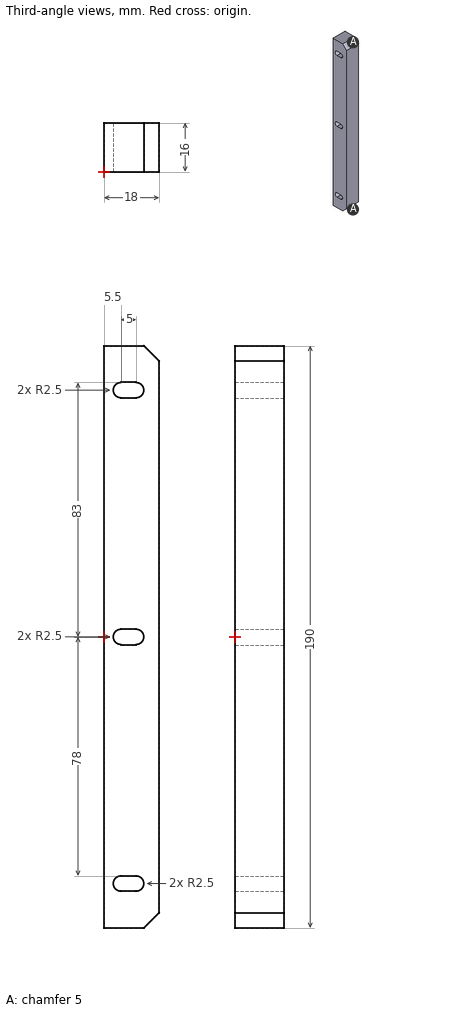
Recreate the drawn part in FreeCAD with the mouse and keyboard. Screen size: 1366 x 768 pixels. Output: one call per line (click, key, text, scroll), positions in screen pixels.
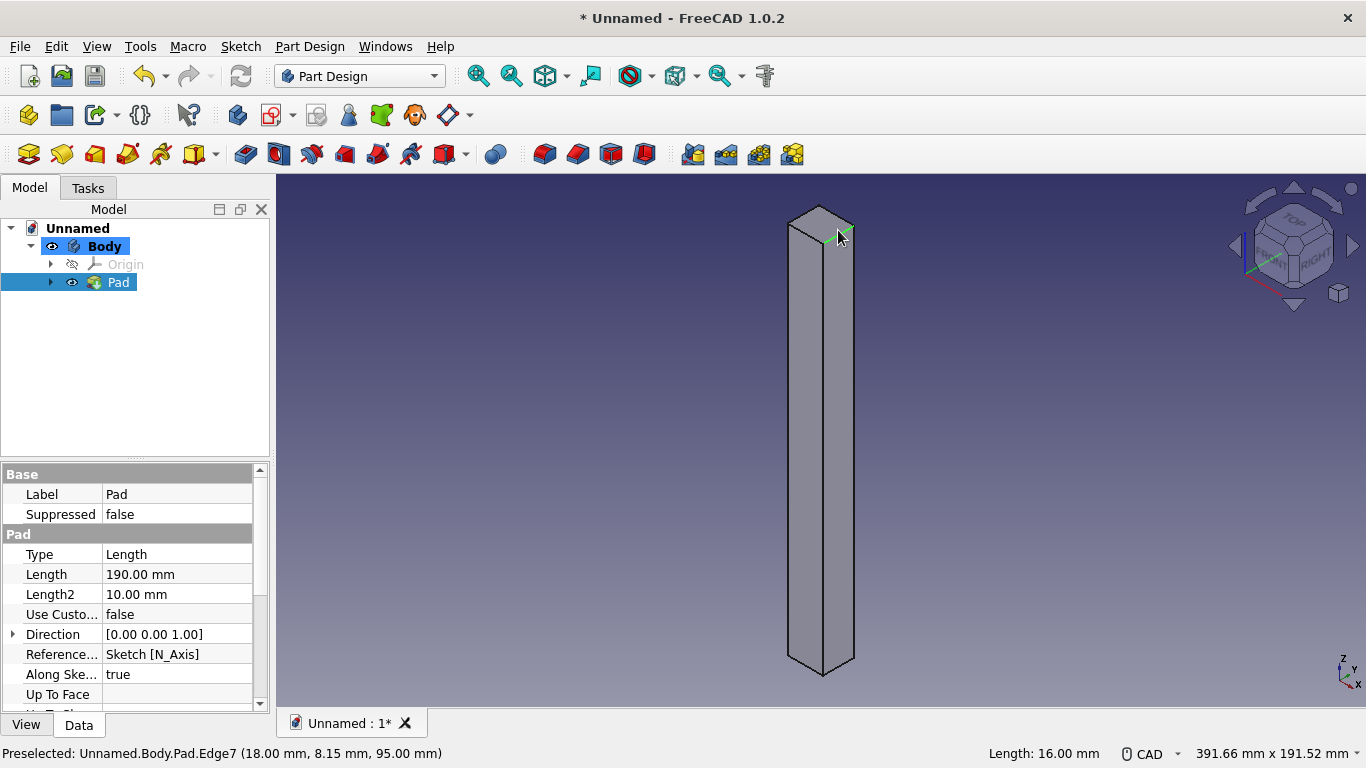
key(2)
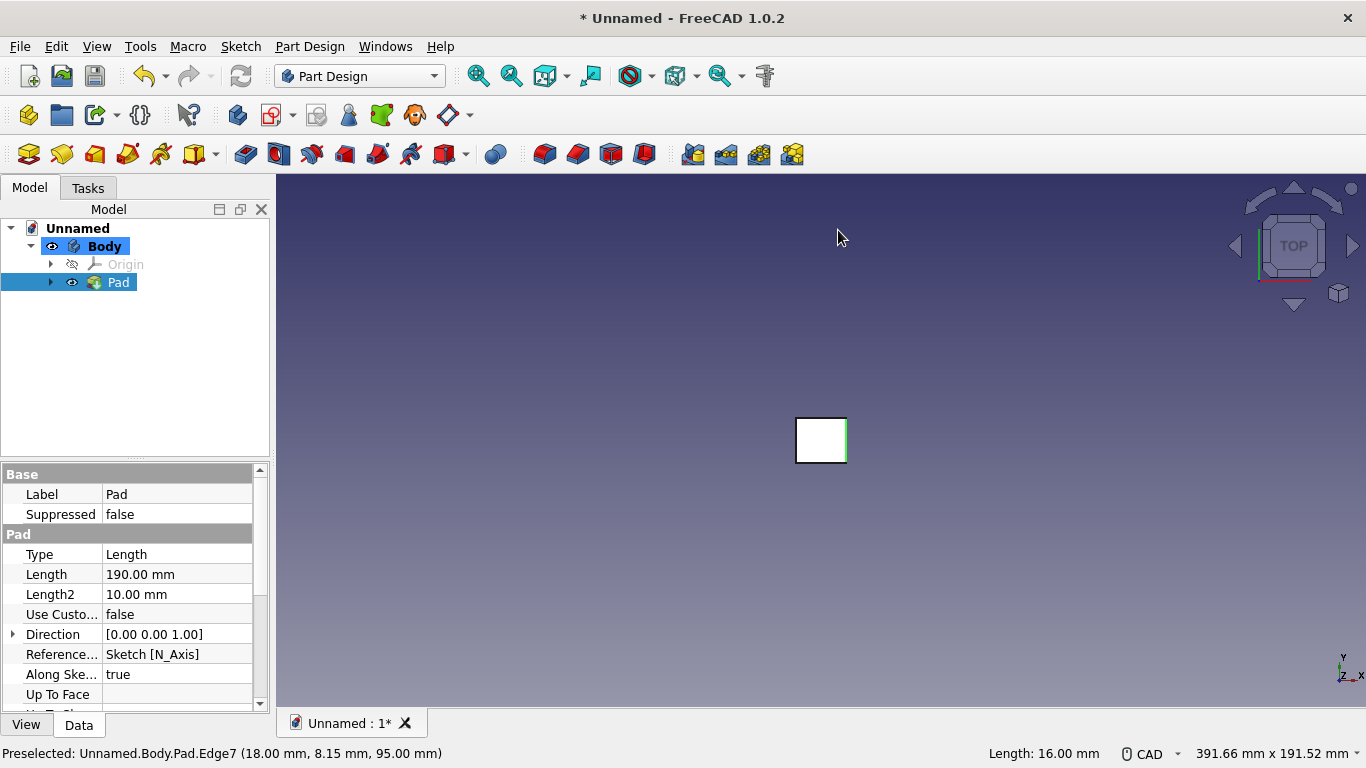
click(479, 76)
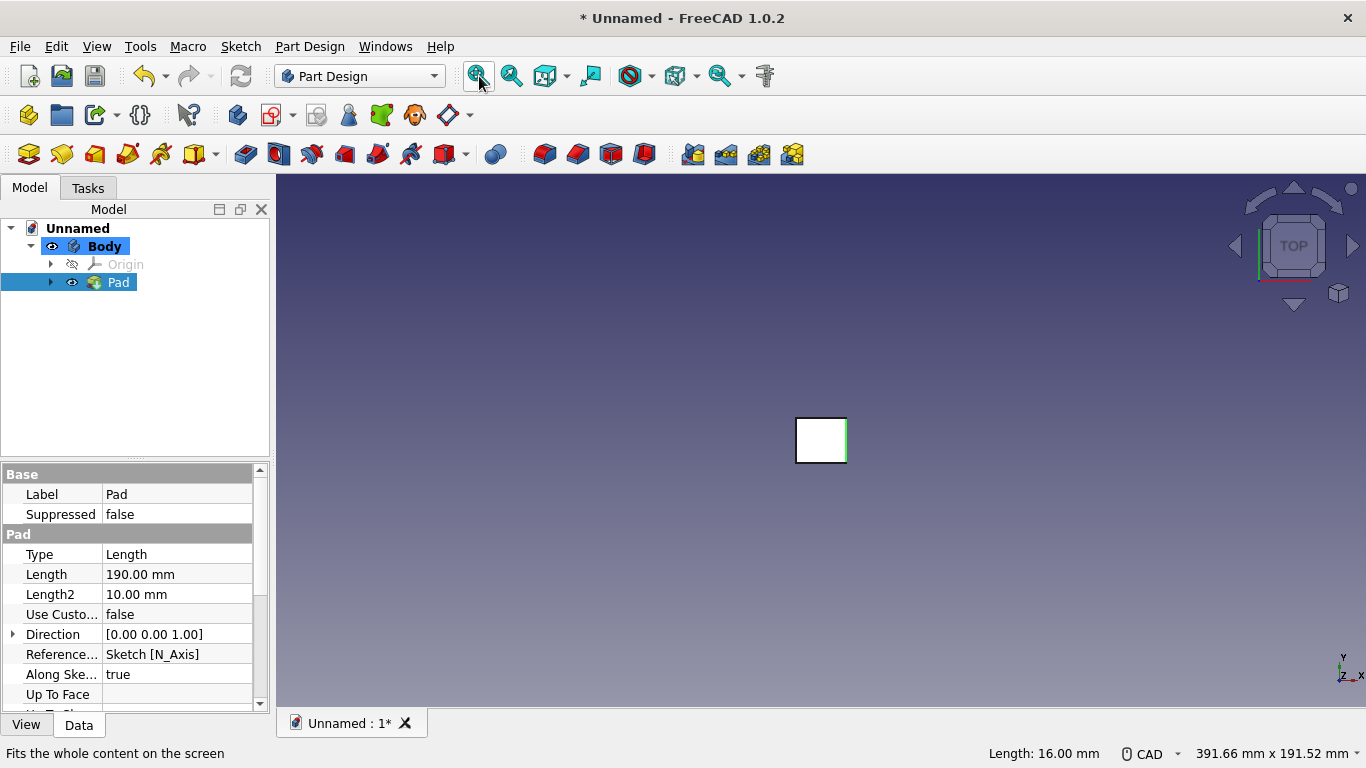
key(1)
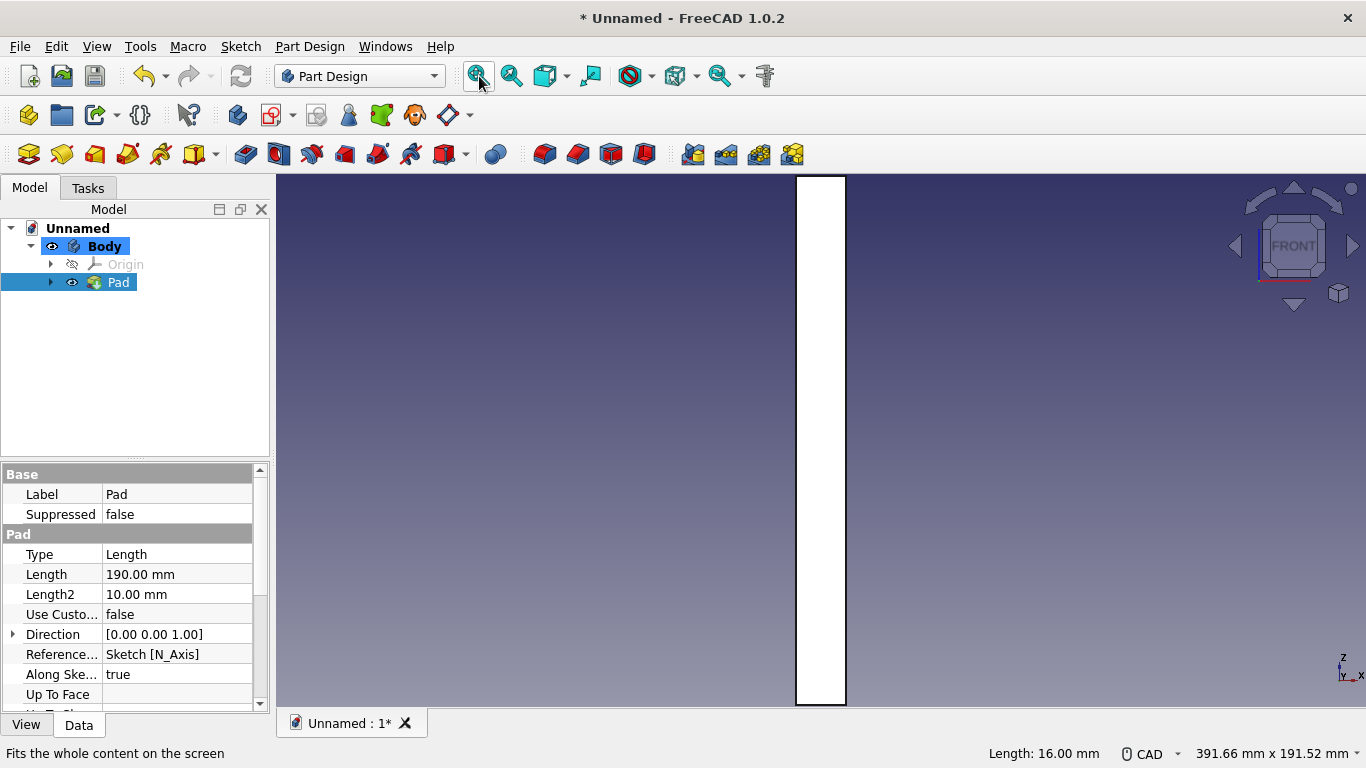
key(3)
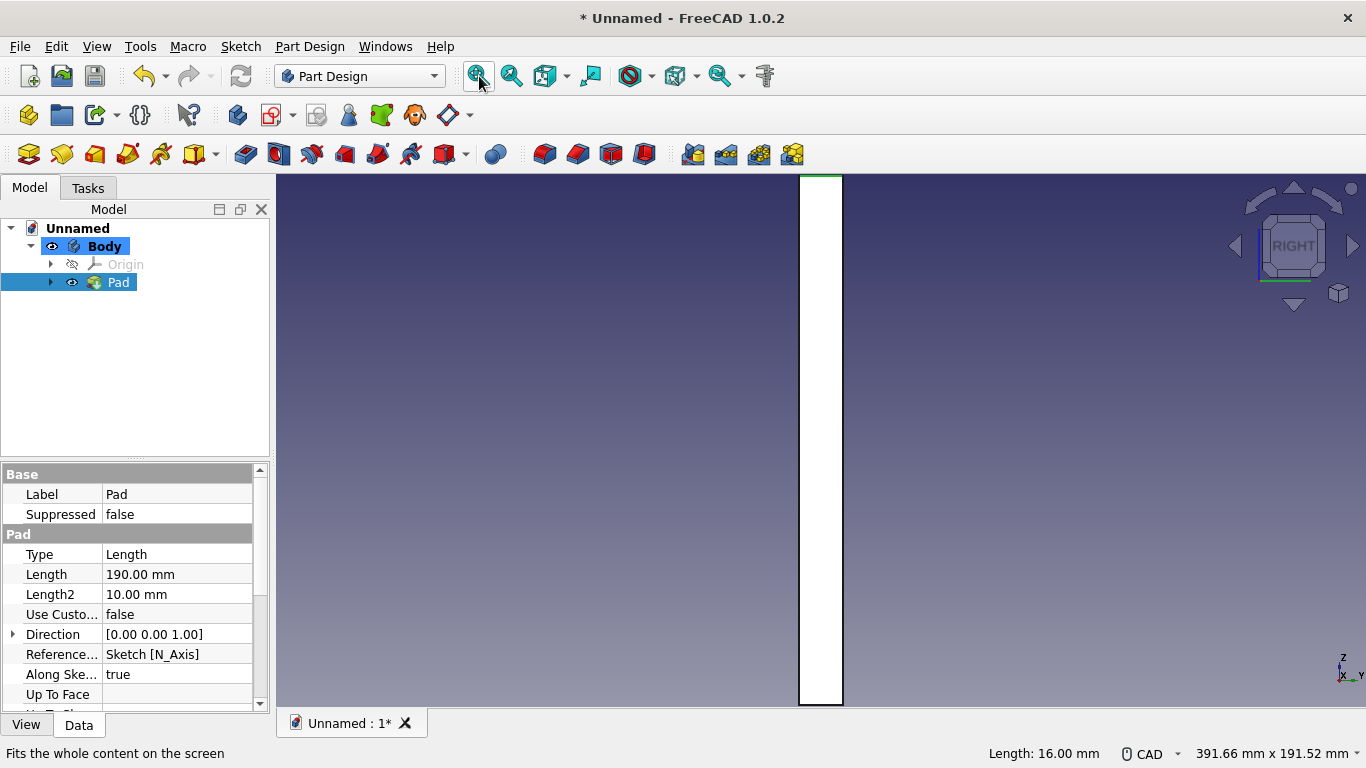
key(5)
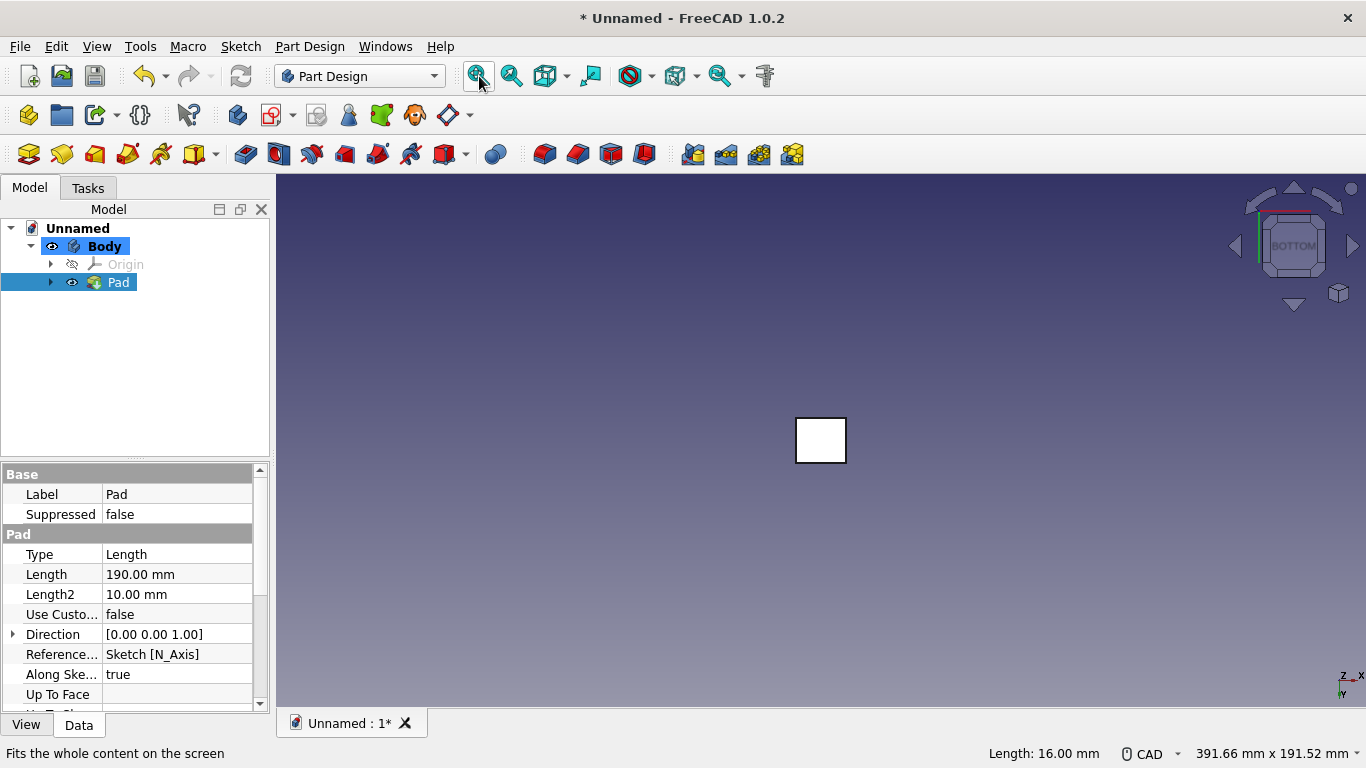
key(v)
key(f)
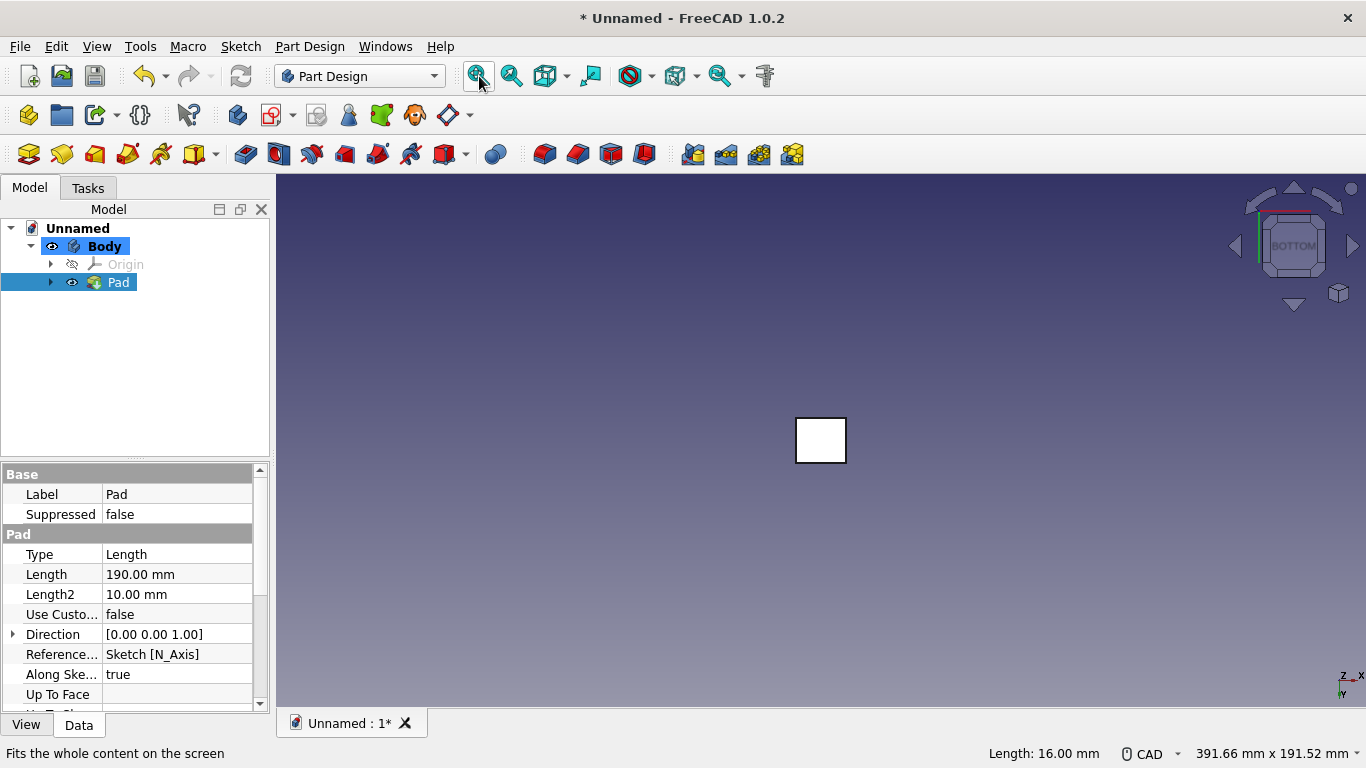
click(846, 439, ctrl)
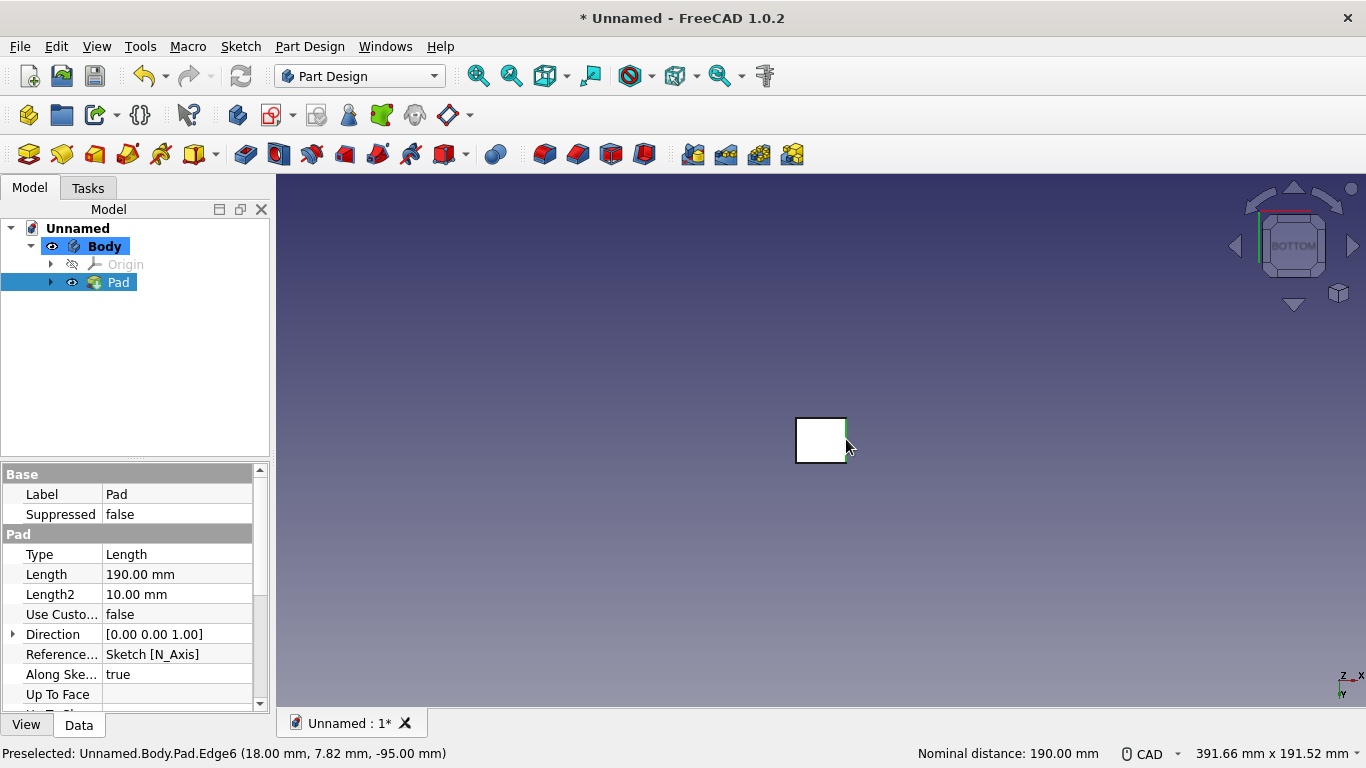
click(578, 154)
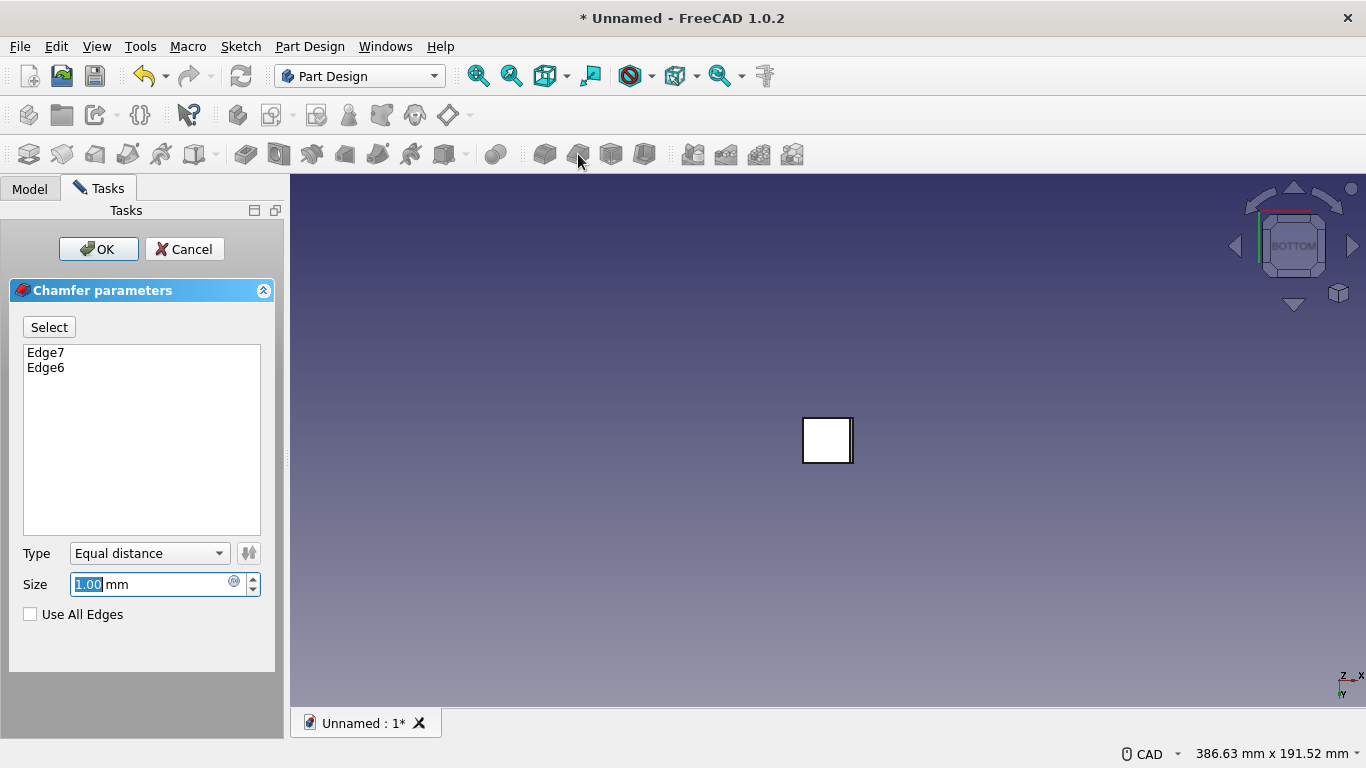
text(5)
key(Tab)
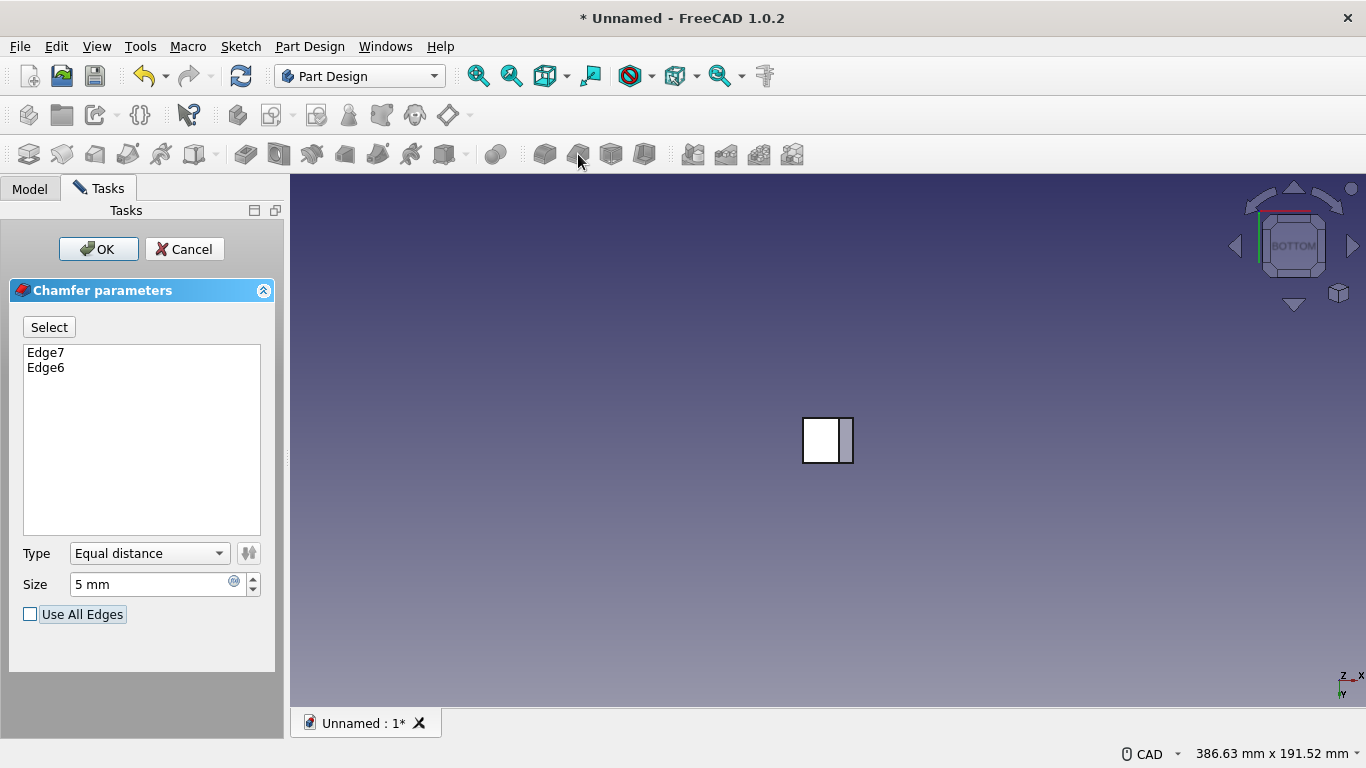
click(99, 249)